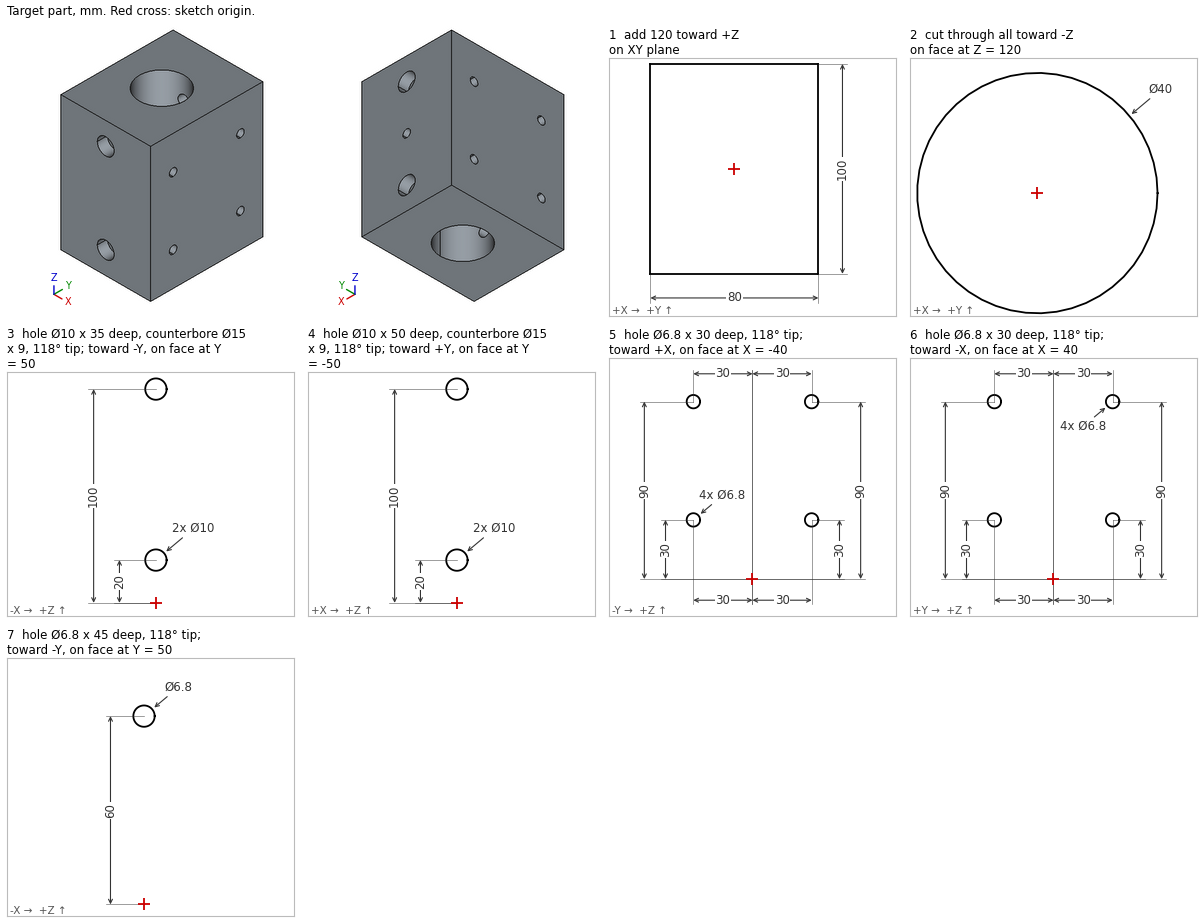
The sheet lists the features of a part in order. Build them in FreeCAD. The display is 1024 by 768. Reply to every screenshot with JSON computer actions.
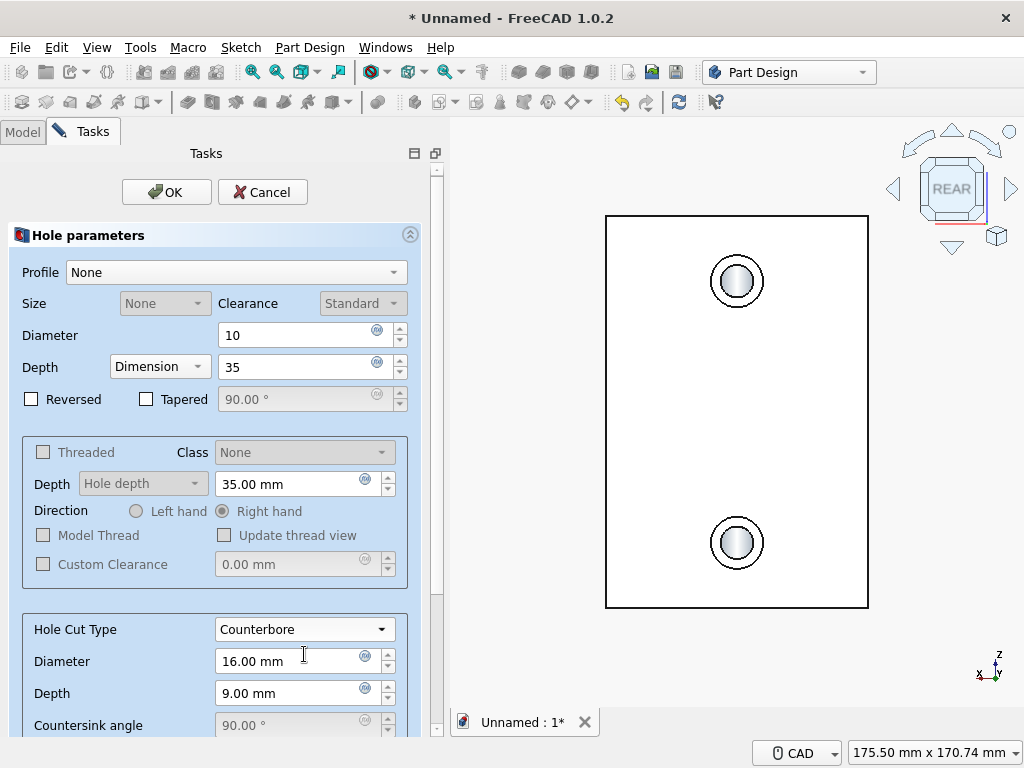
{"action": "triple_click", "coordinate": [298, 661]}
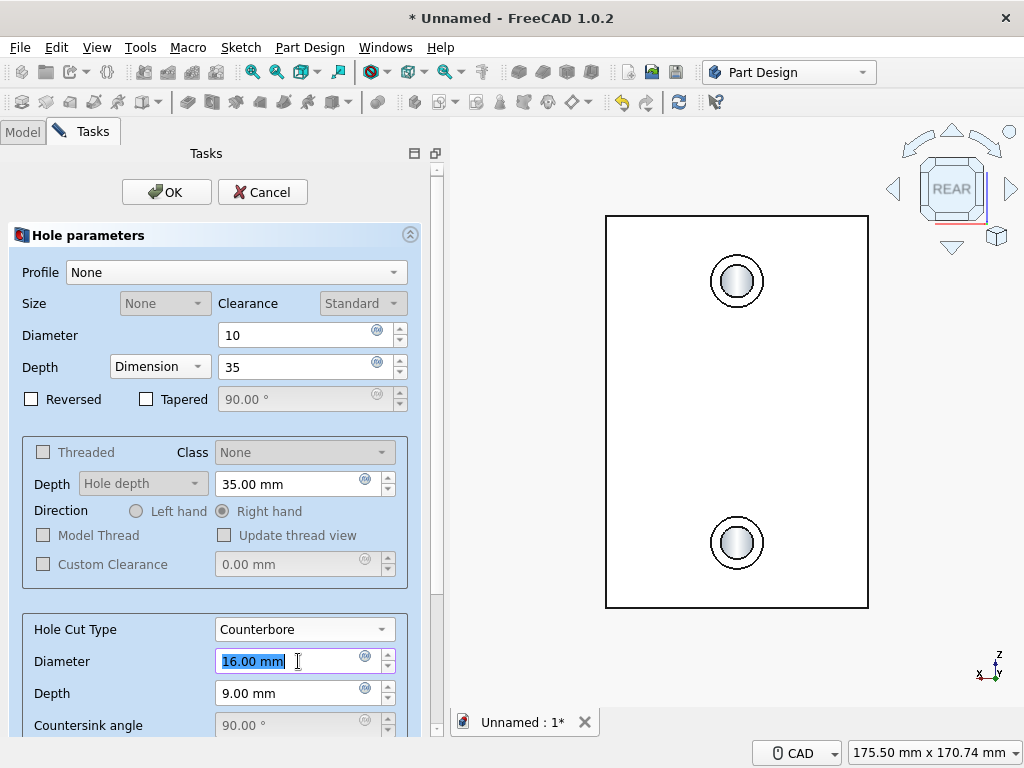
{"action": "type", "text": "15"}
{"action": "key", "text": "Tab"}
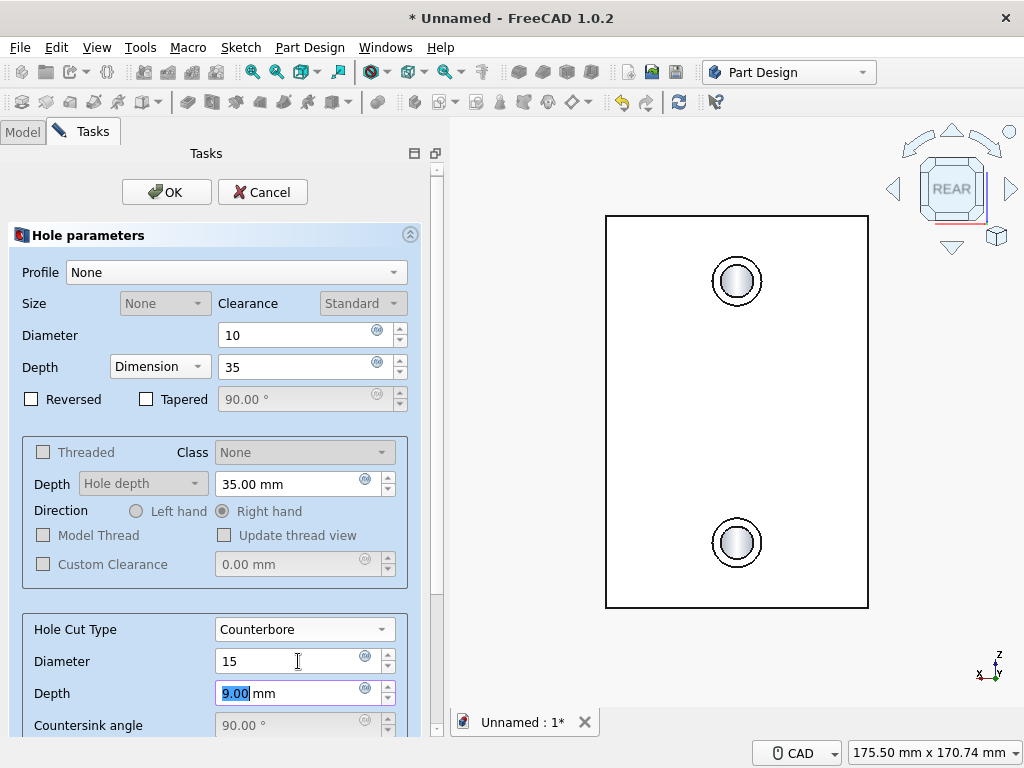
{"action": "type", "text": "9"}
{"action": "key", "text": "Tab"}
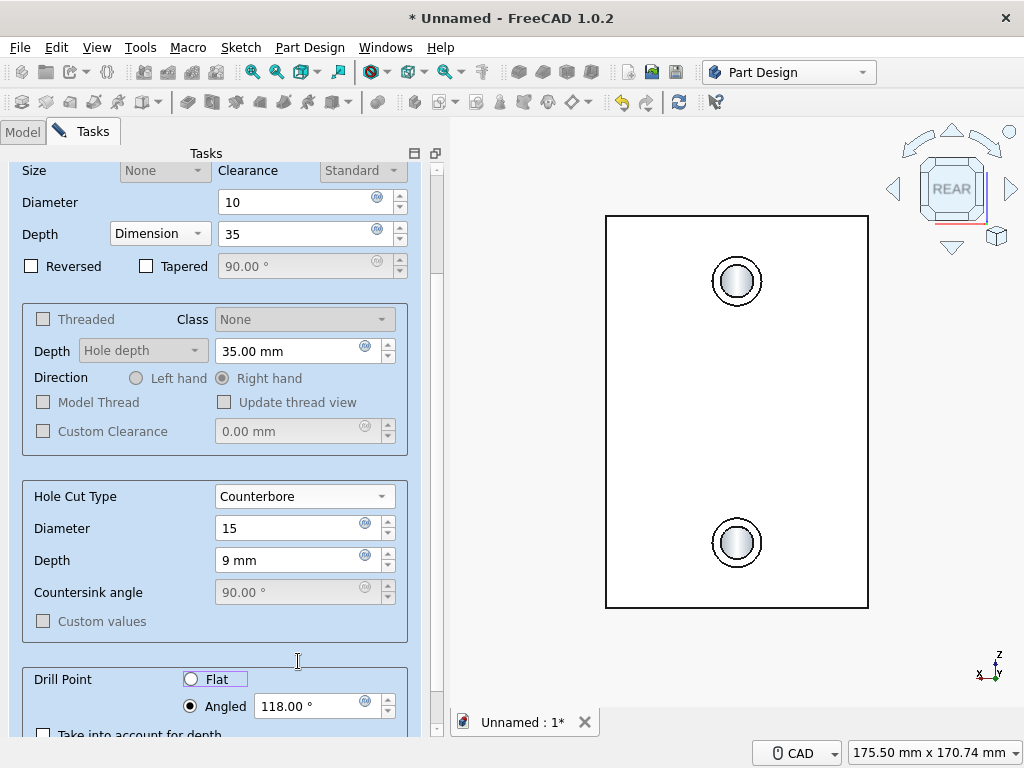
{"action": "scroll", "coordinate": [437, 450], "scroll_direction": "up", "scroll_amount": 3}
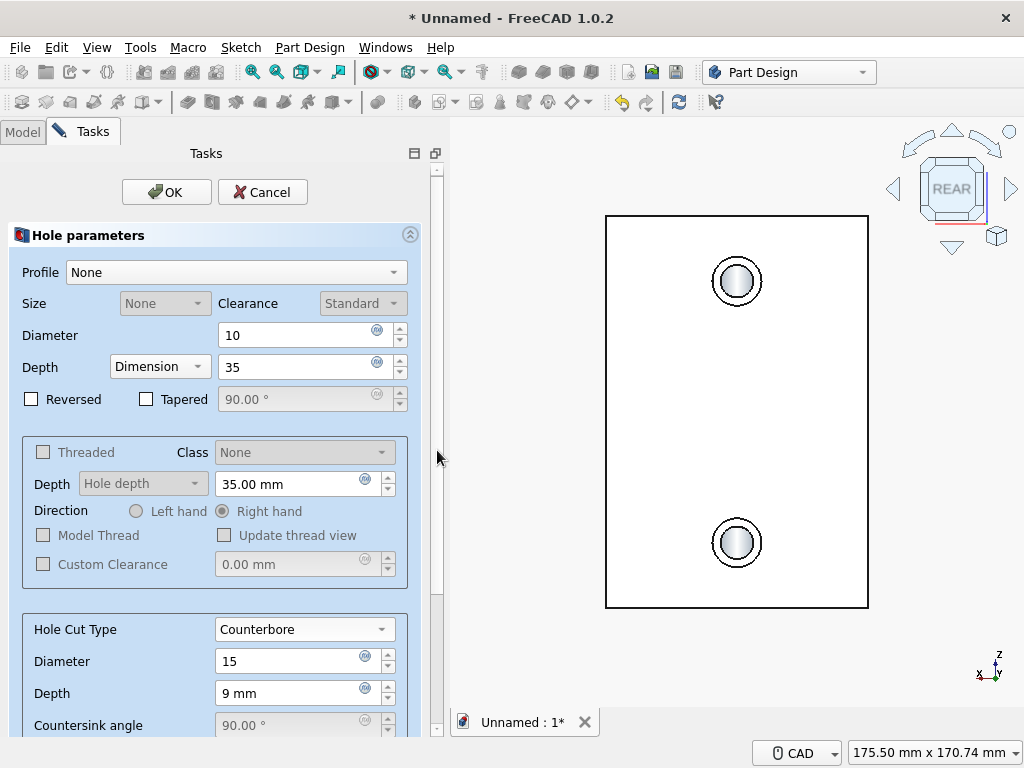
{"action": "left_click", "coordinate": [167, 192]}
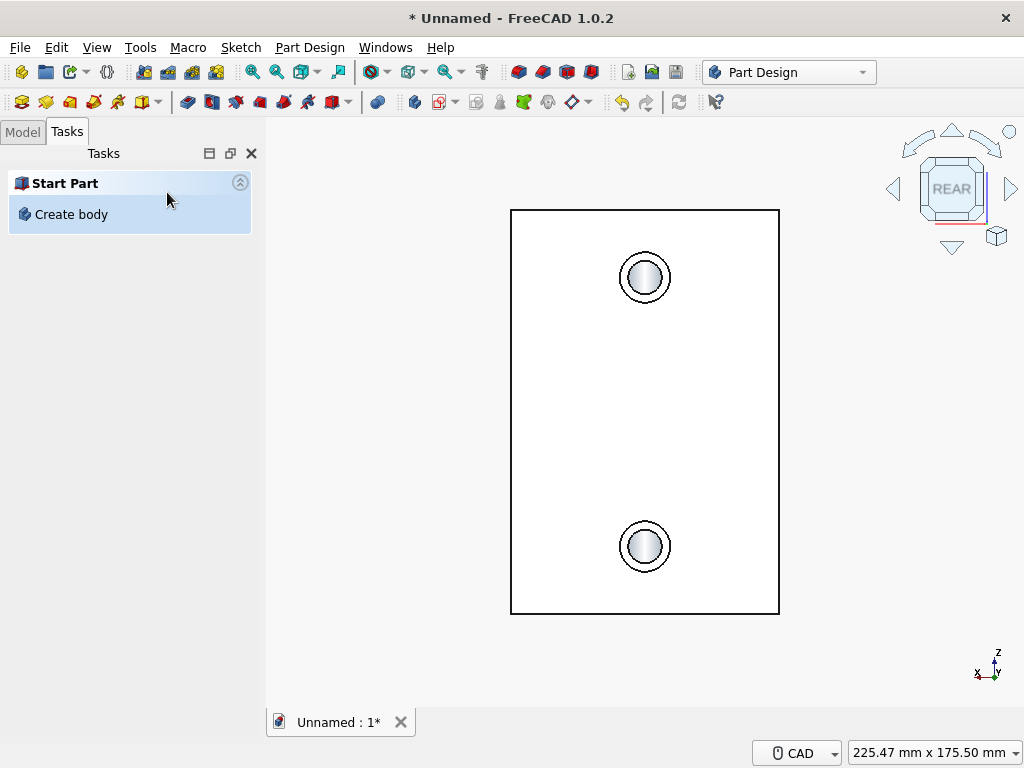
{"action": "key", "text": "0"}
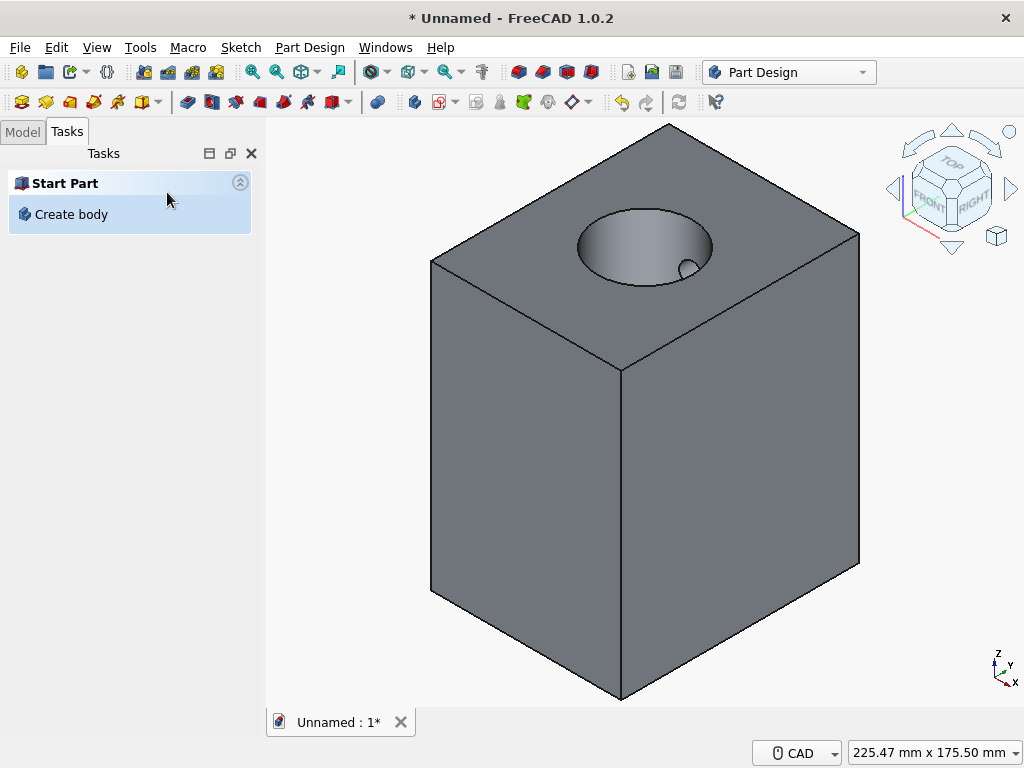
{"action": "left_click", "coordinate": [526, 433]}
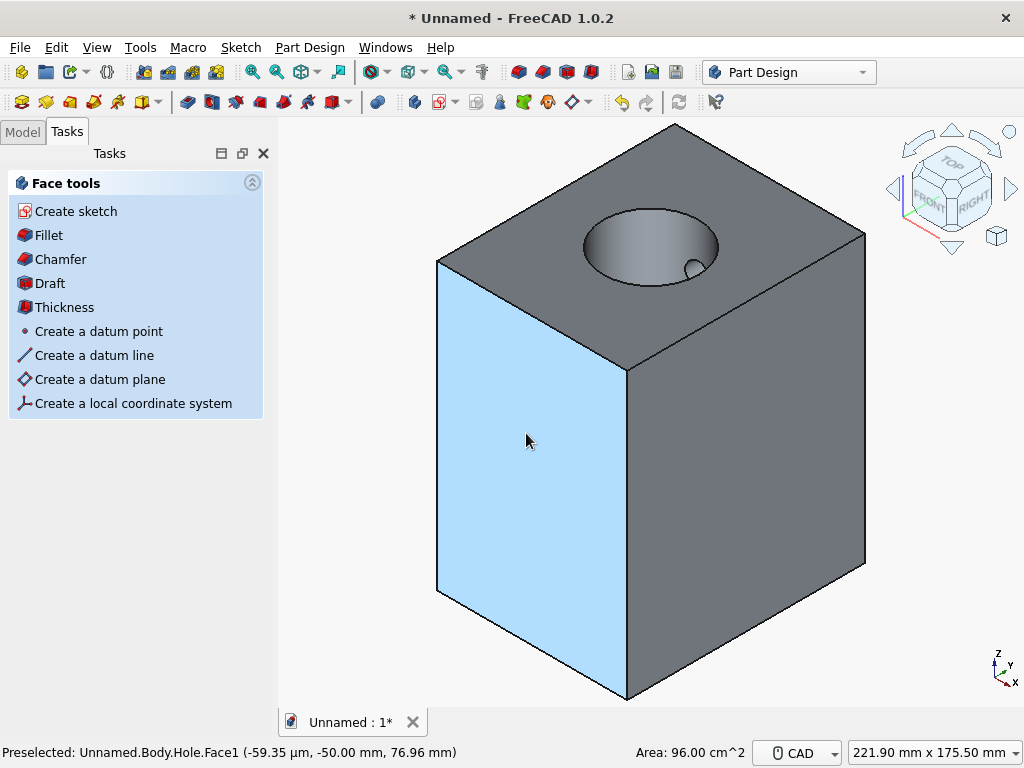
{"action": "left_click", "coordinate": [440, 102]}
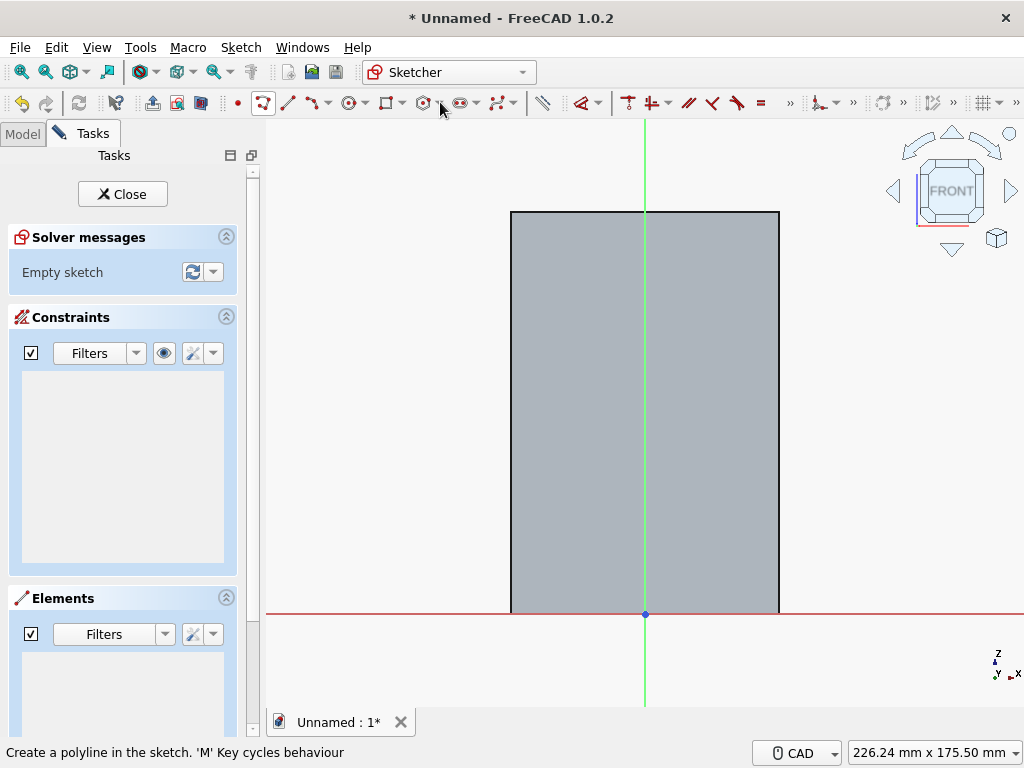
{"action": "left_click", "coordinate": [350, 104]}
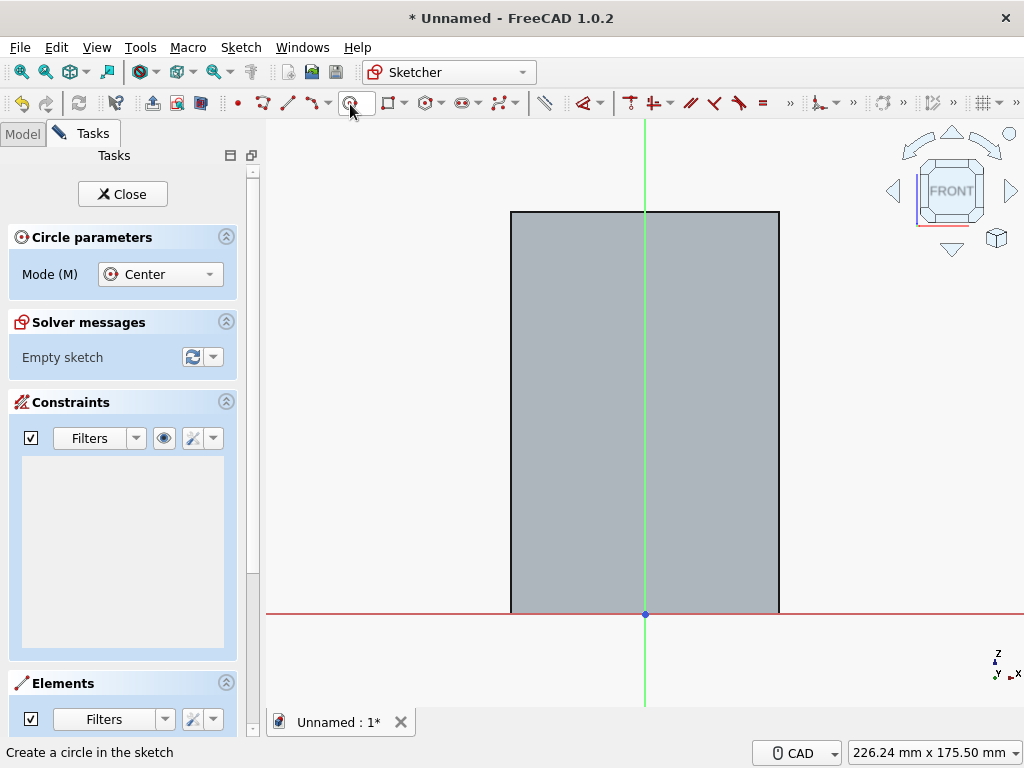
{"action": "scroll", "coordinate": [645, 547], "scroll_direction": "up", "scroll_amount": 2}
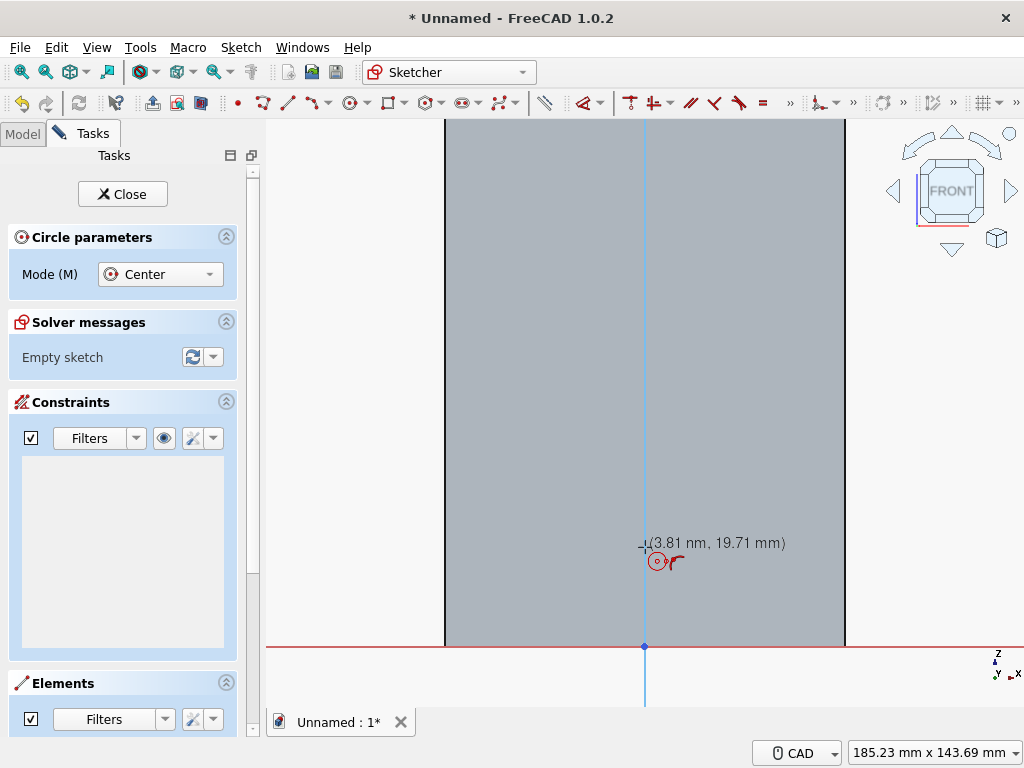
{"action": "left_click", "coordinate": [645, 547]}
{"action": "mouse_move", "coordinate": [662, 529]}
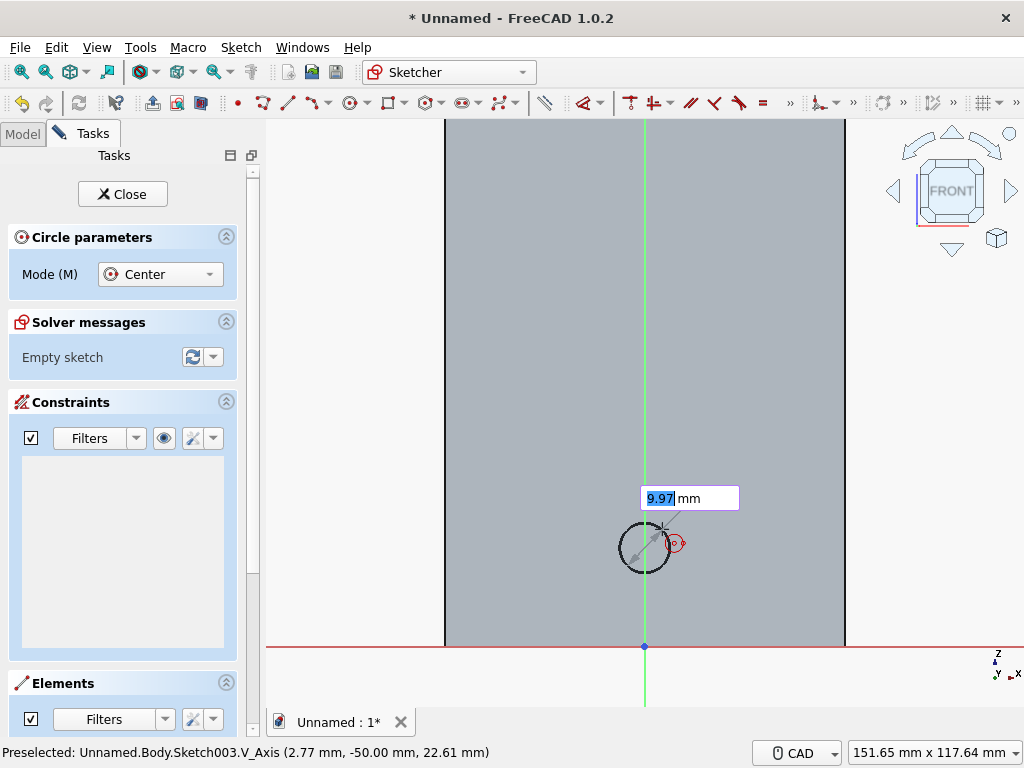
{"action": "type", "text": "10"}
{"action": "key", "text": "Return"}